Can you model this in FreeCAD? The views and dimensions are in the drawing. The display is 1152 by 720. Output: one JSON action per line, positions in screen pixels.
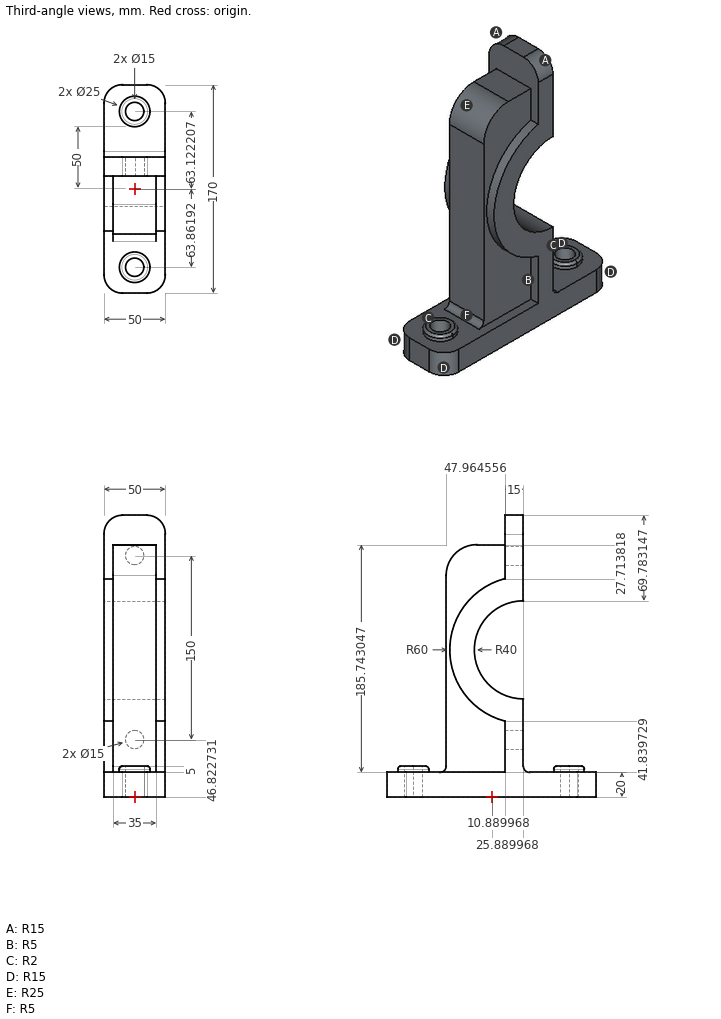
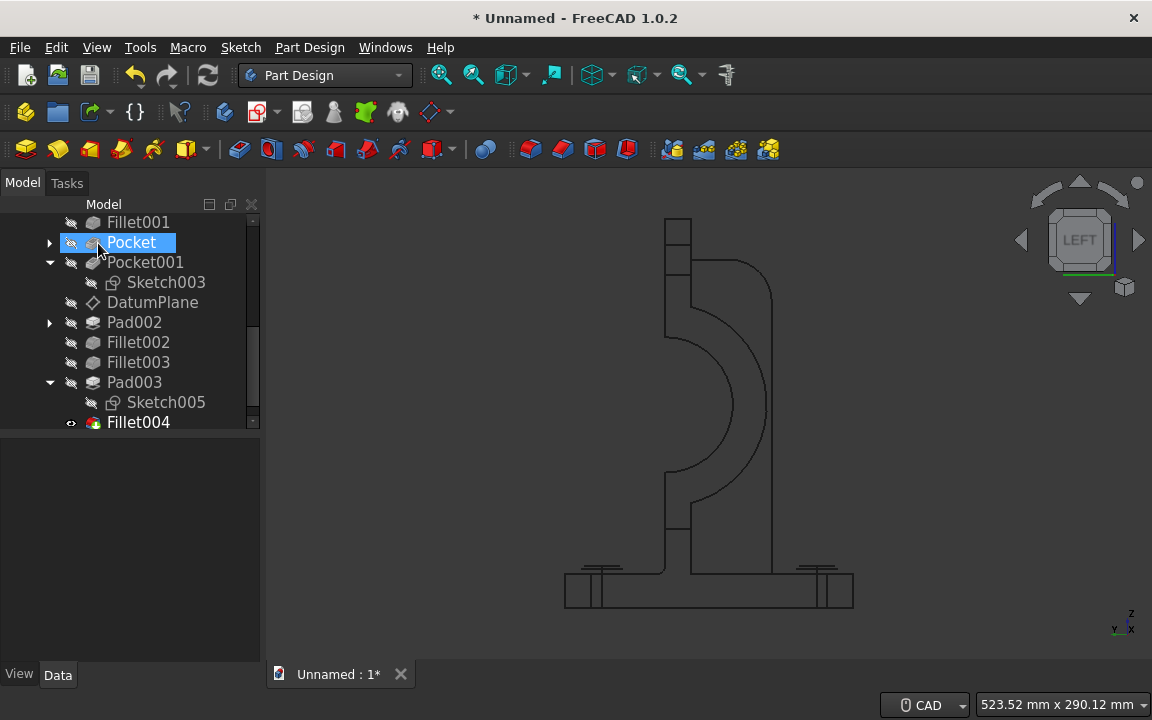
{"action": "key", "text": "0"}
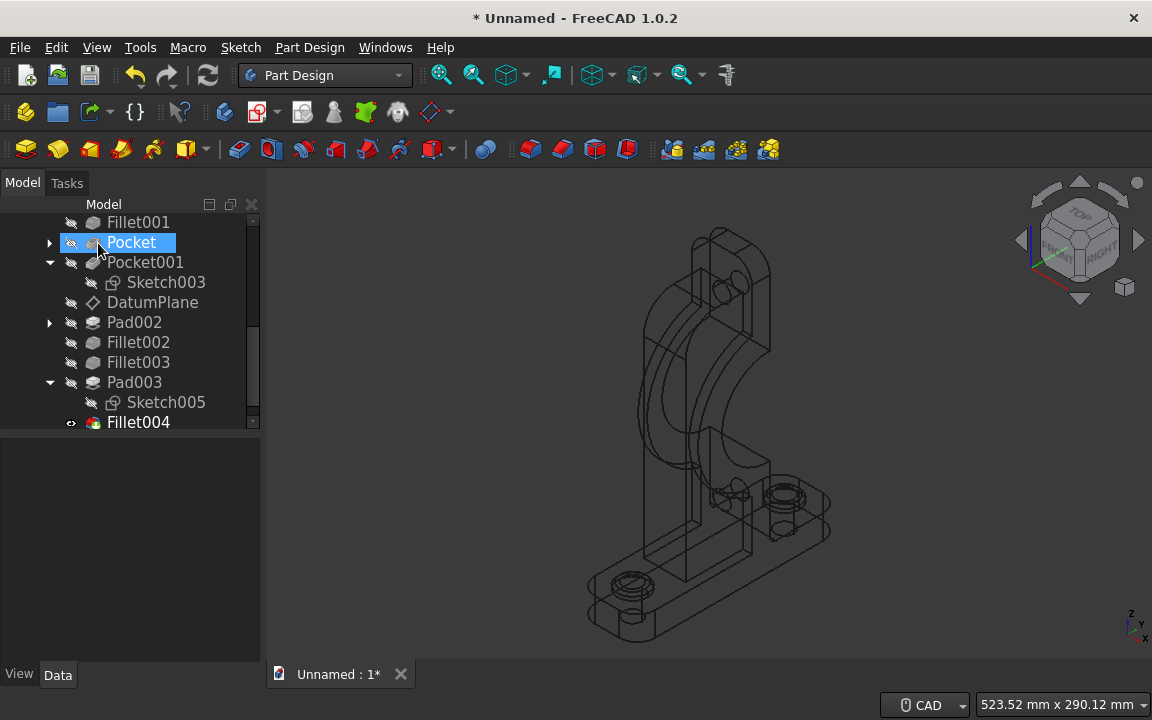
{"action": "left_click", "coordinate": [665, 569]}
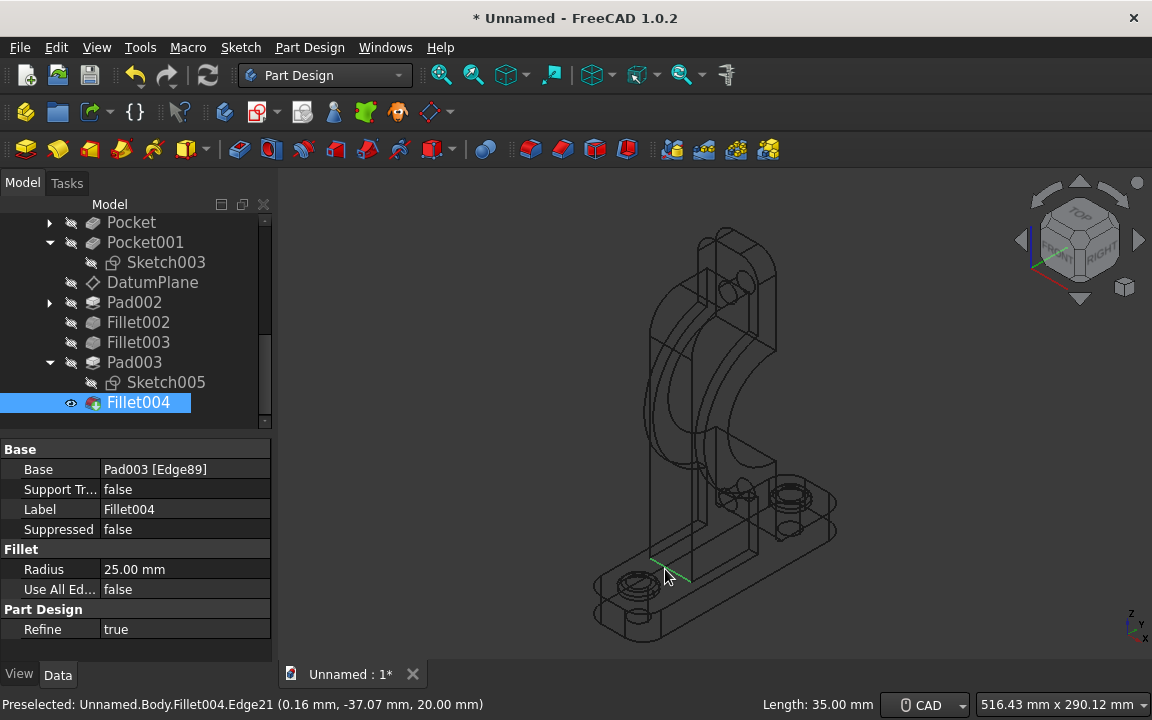
{"action": "key", "text": "v 1"}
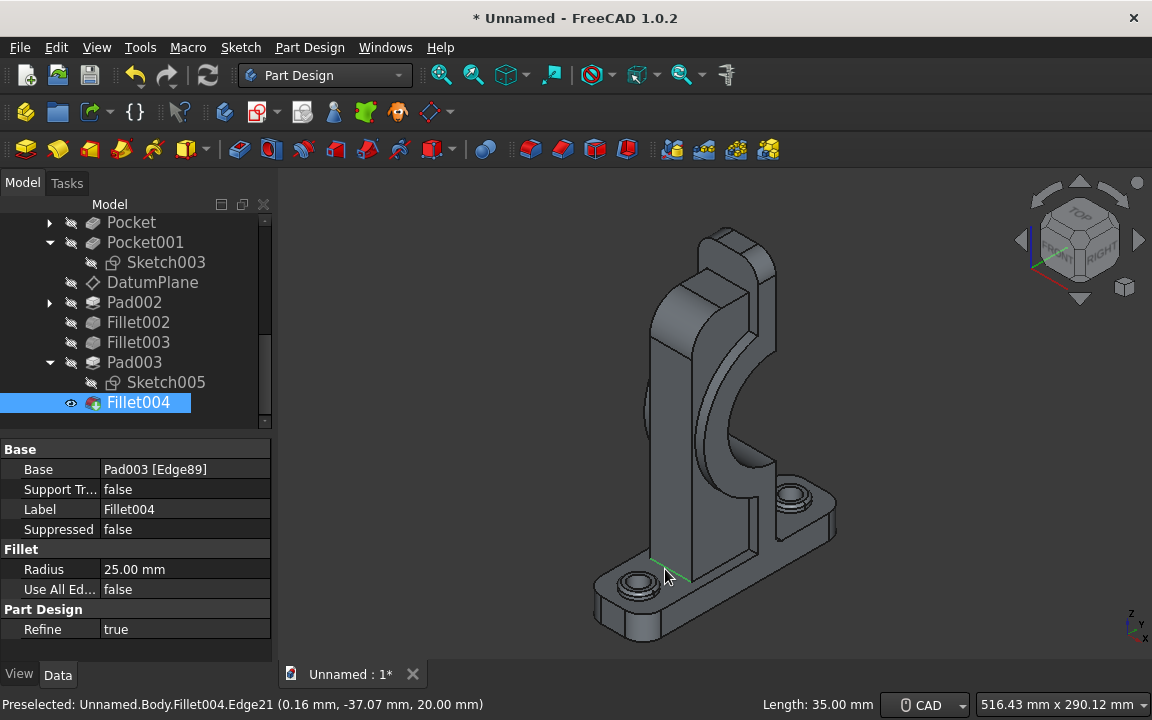
{"action": "left_click", "coordinate": [532, 150]}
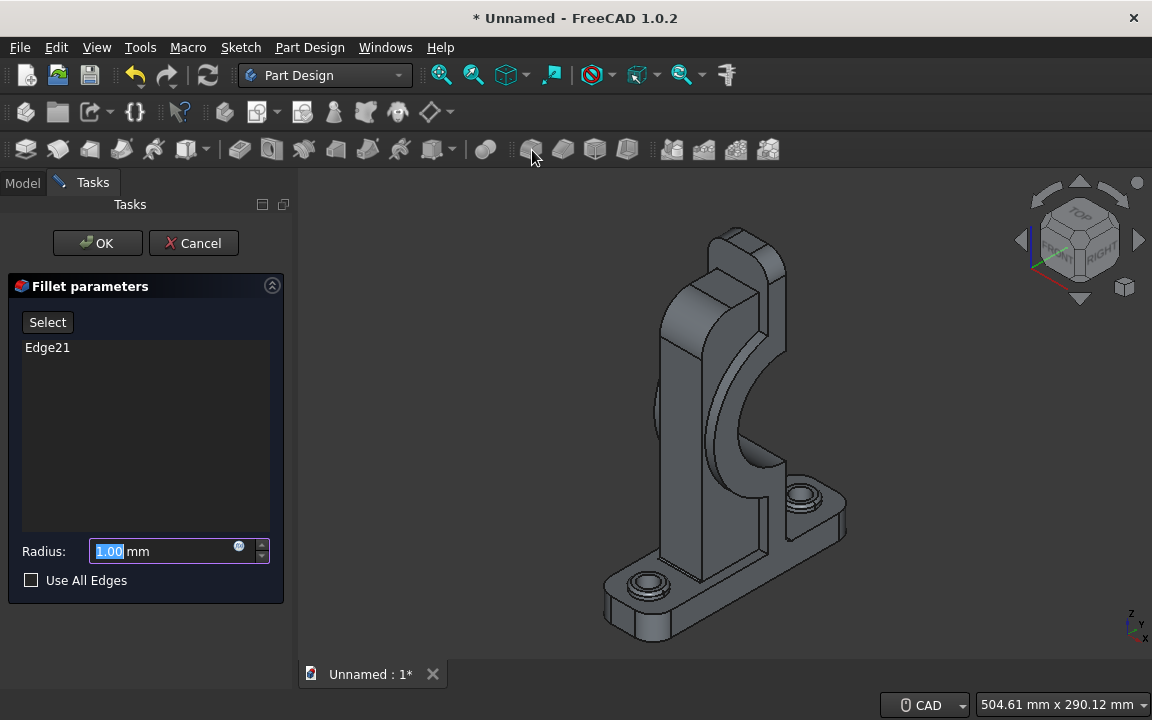
{"action": "type", "text": "5"}
{"action": "key", "text": "Tab"}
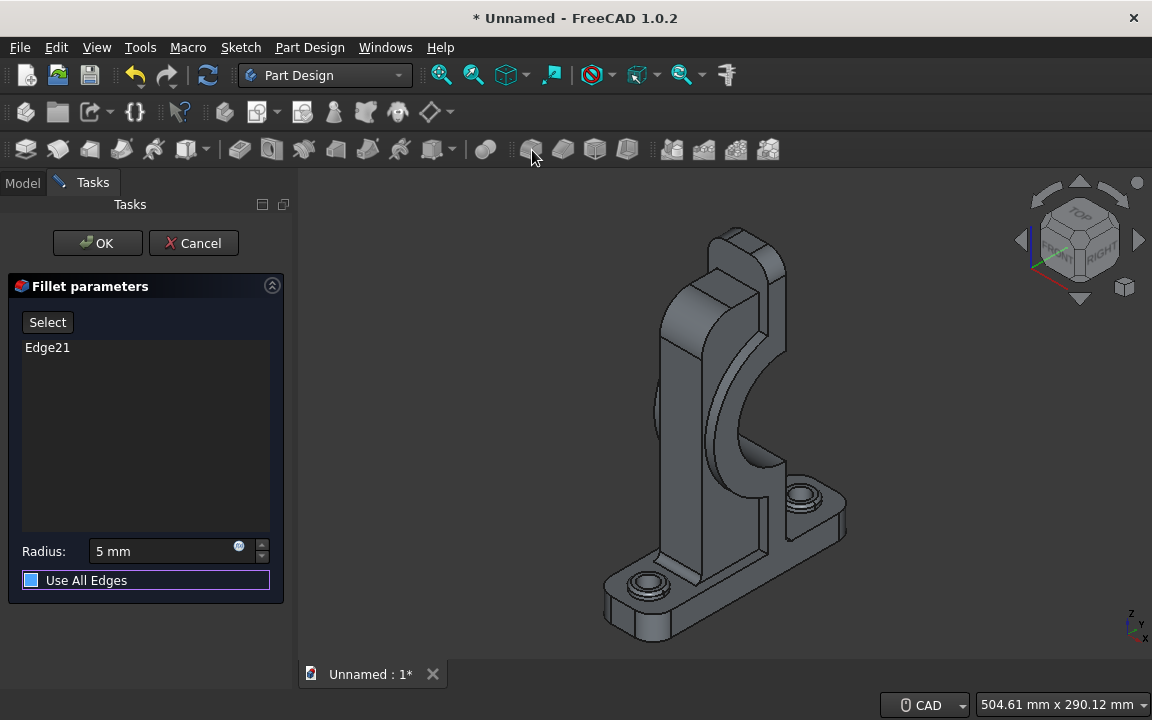
{"action": "left_click", "coordinate": [98, 243]}